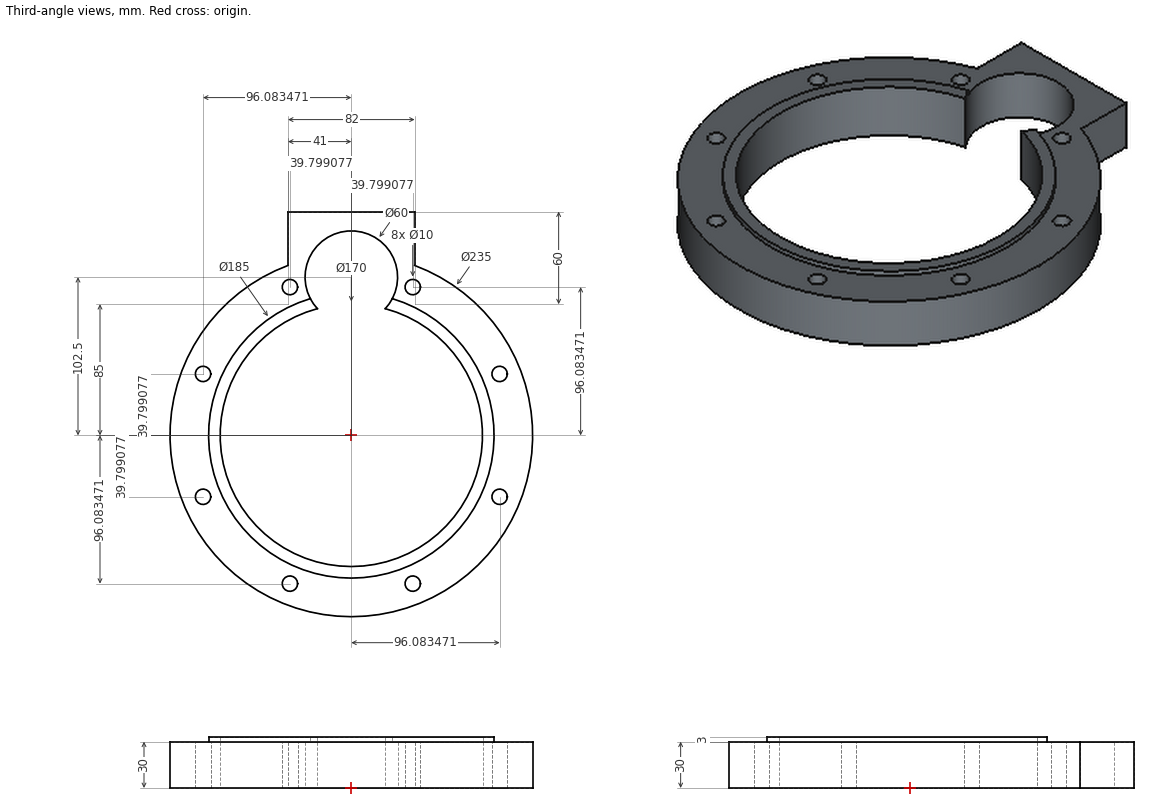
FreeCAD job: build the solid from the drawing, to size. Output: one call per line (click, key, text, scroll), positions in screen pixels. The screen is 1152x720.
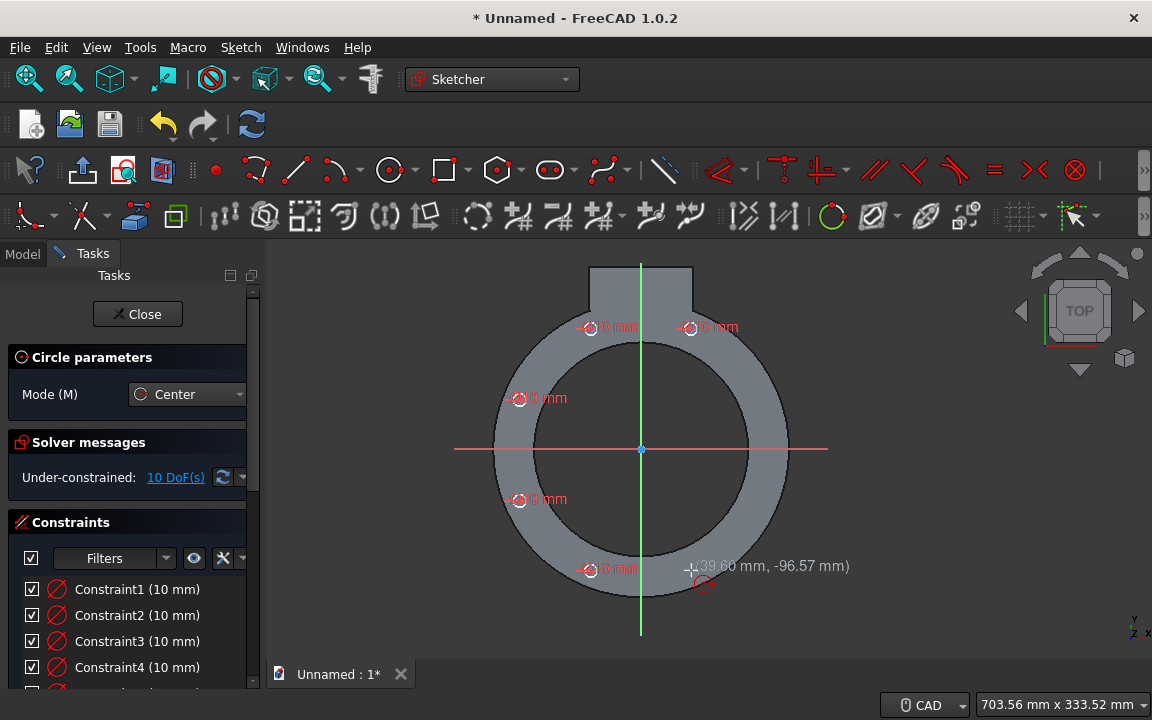
click(691, 570)
move(696, 566)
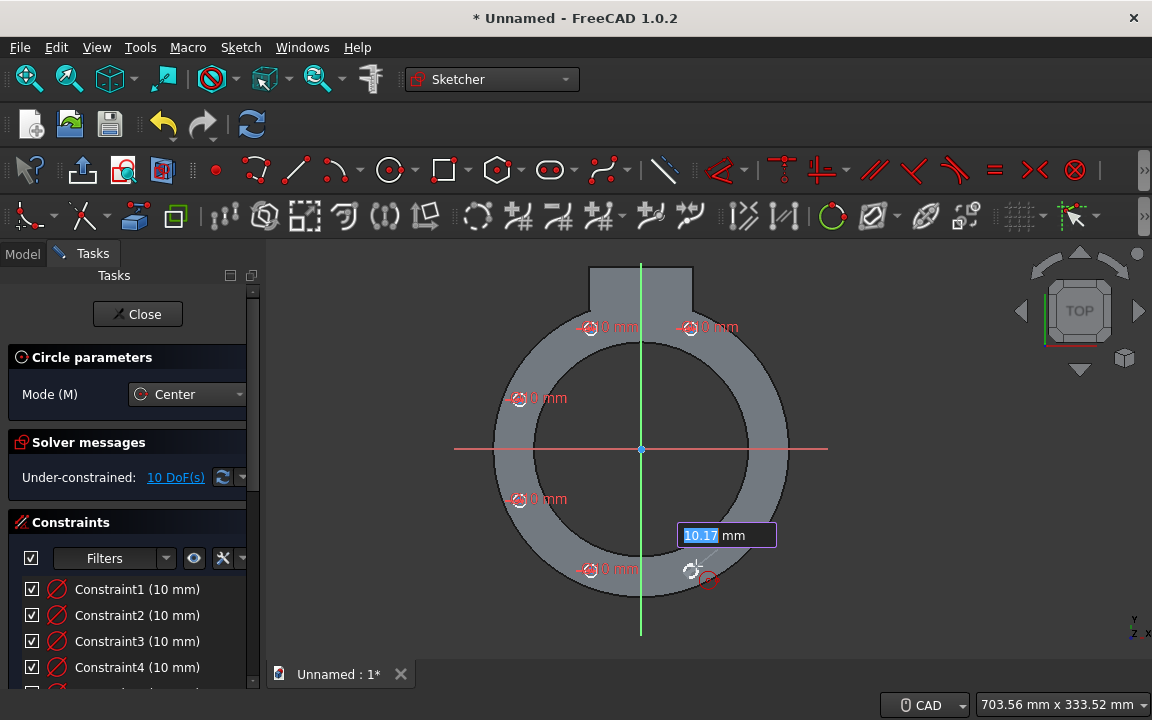
text(10)
key(Return)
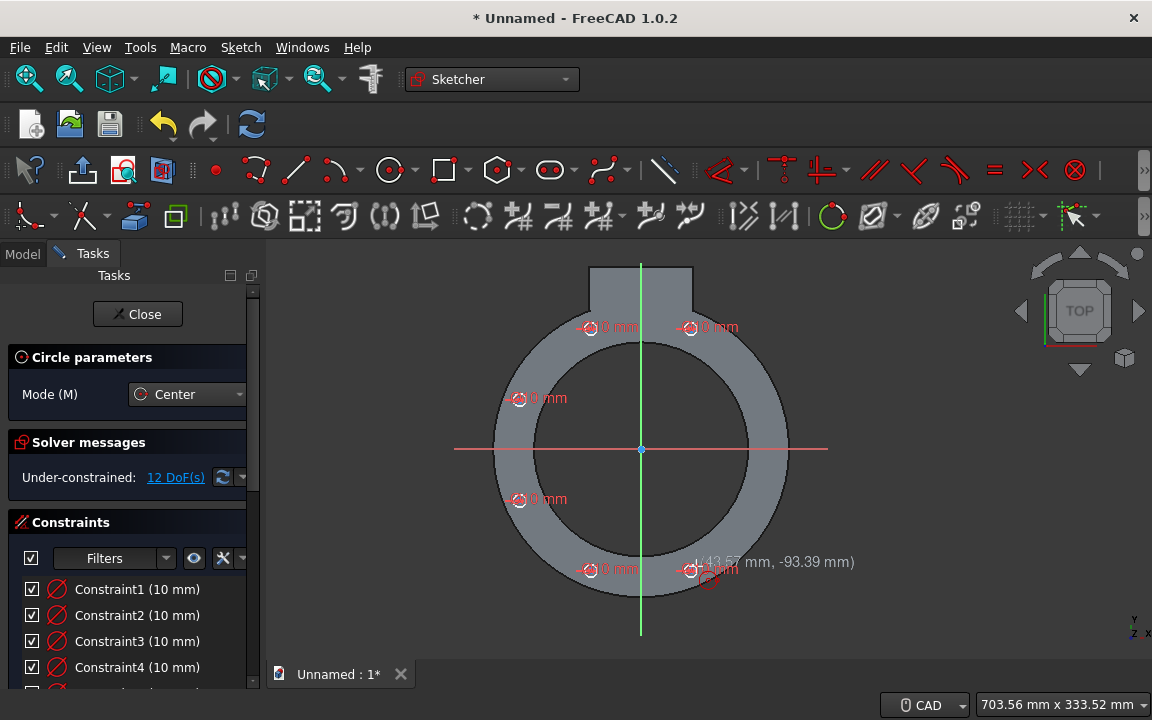
scroll(762, 500, up, 7)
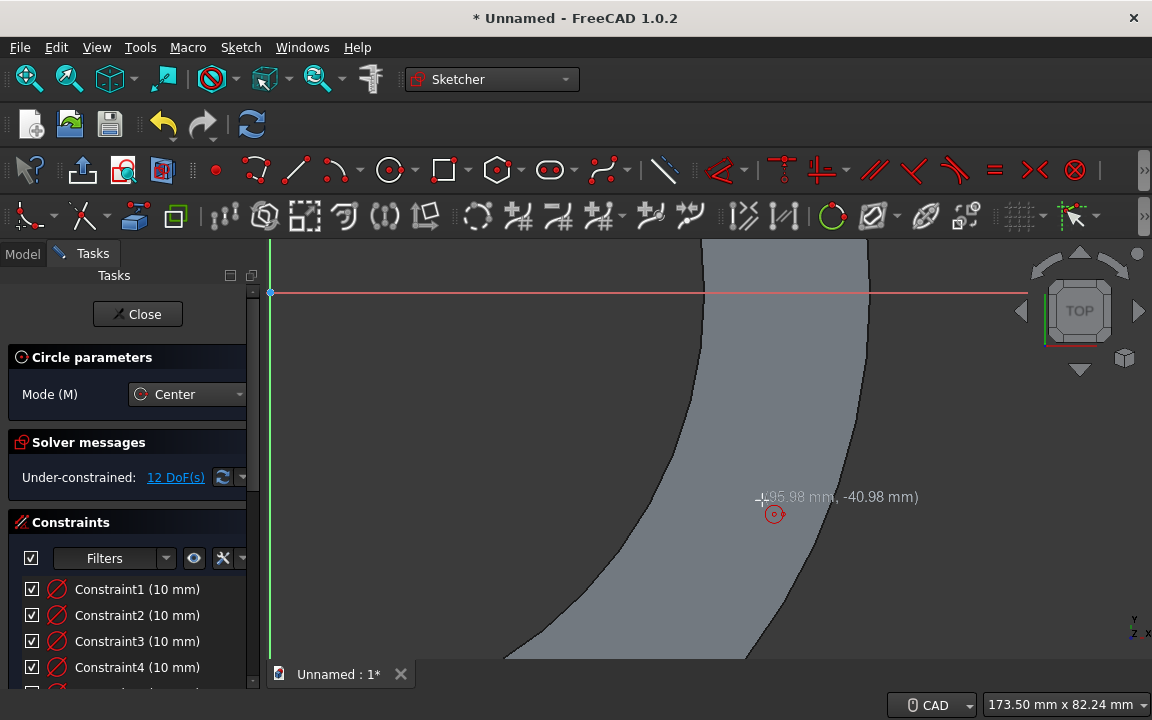
scroll(762, 500, down, 7)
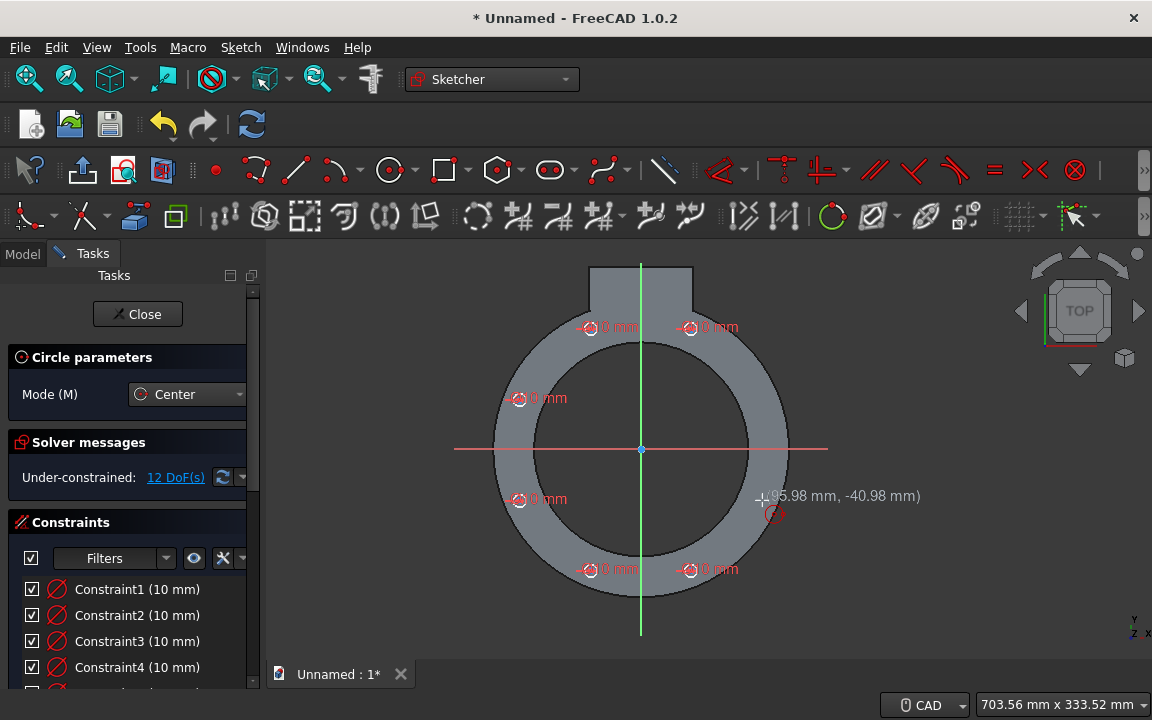
click(762, 500)
move(767, 495)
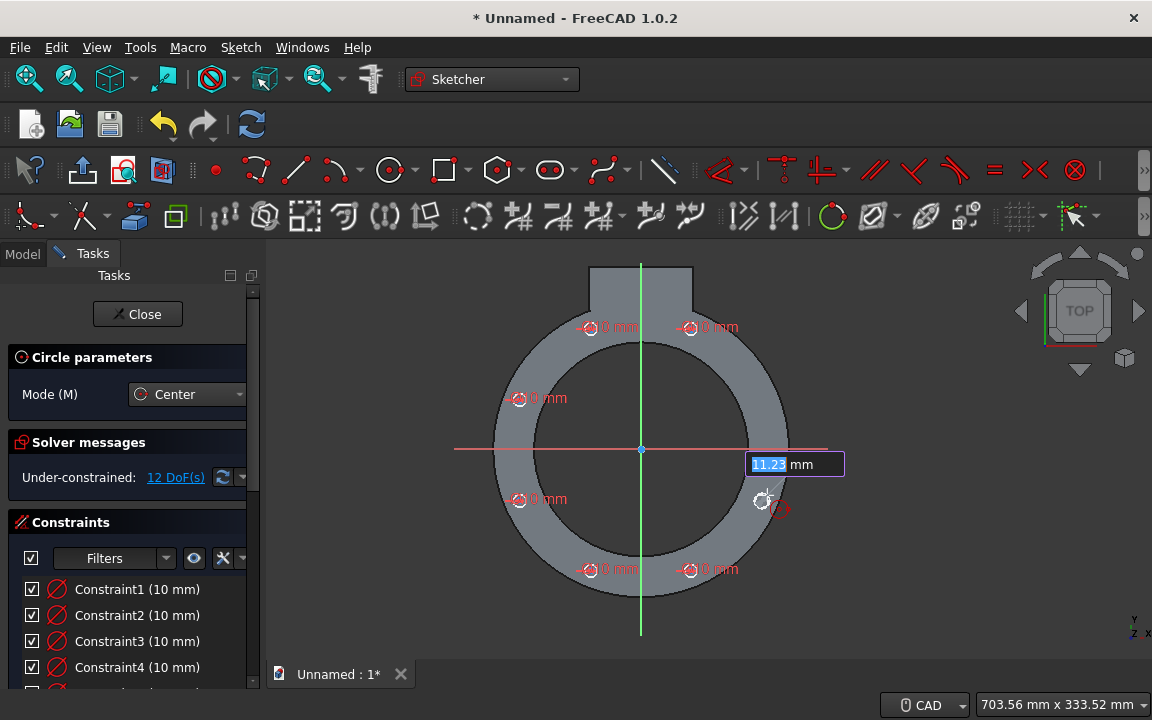
text(10)
key(Return)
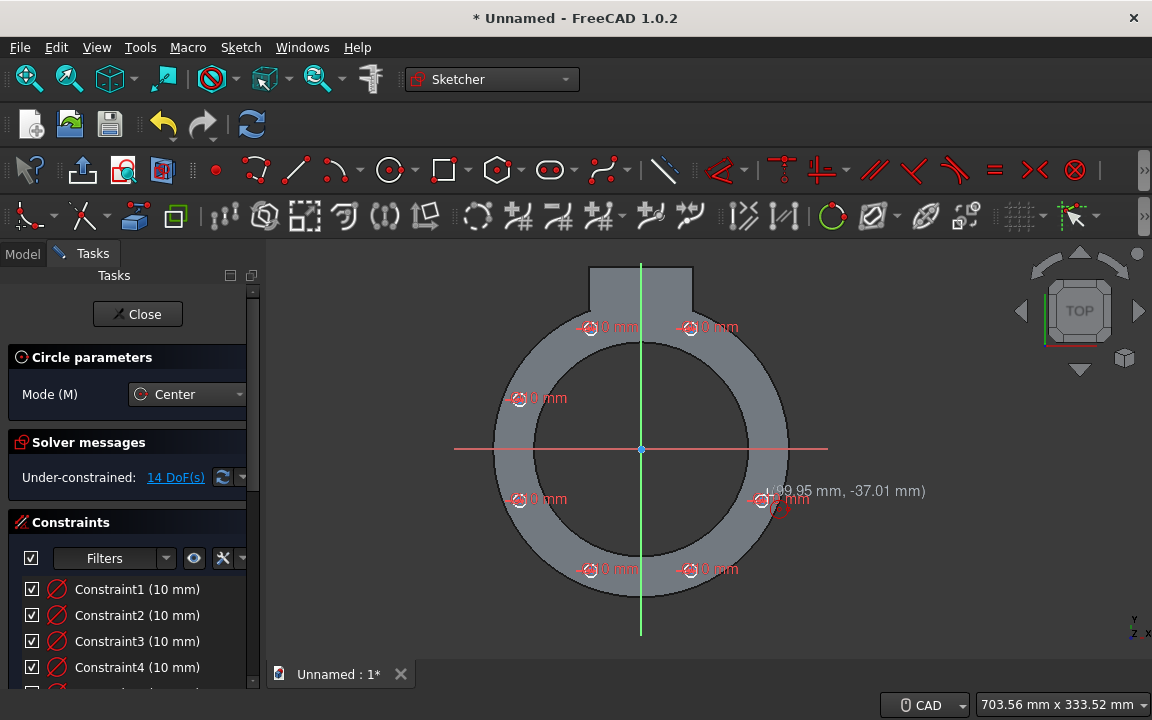
scroll(762, 399, up, 7)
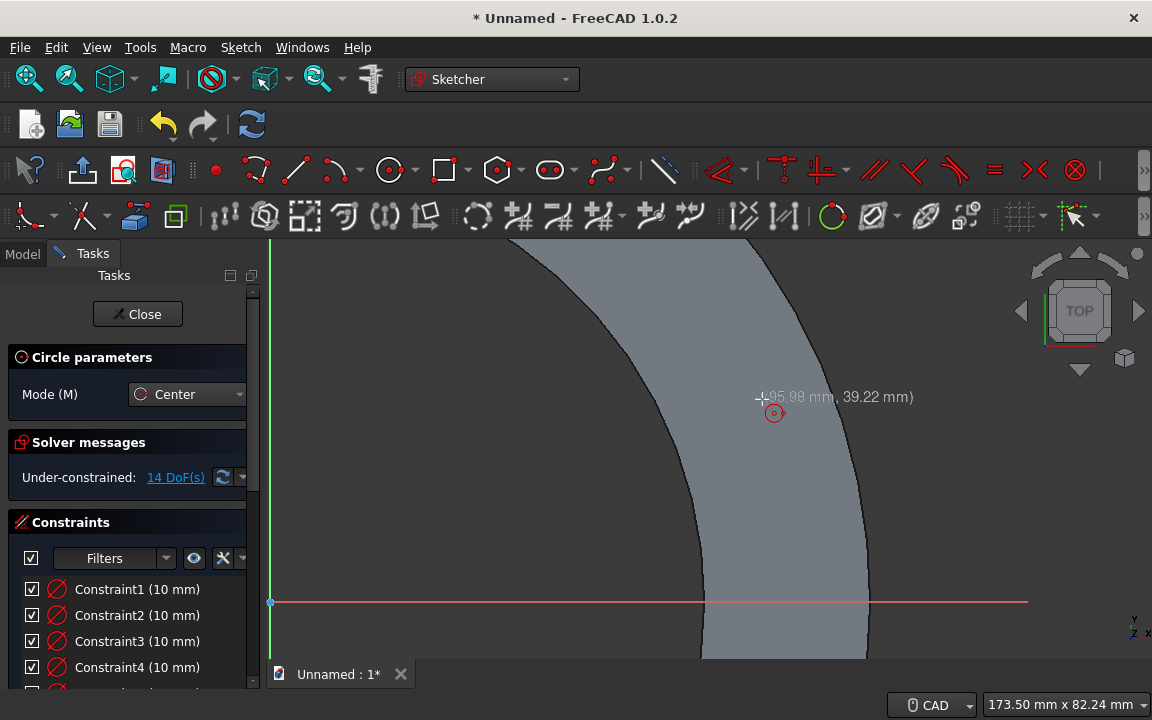
scroll(762, 399, down, 7)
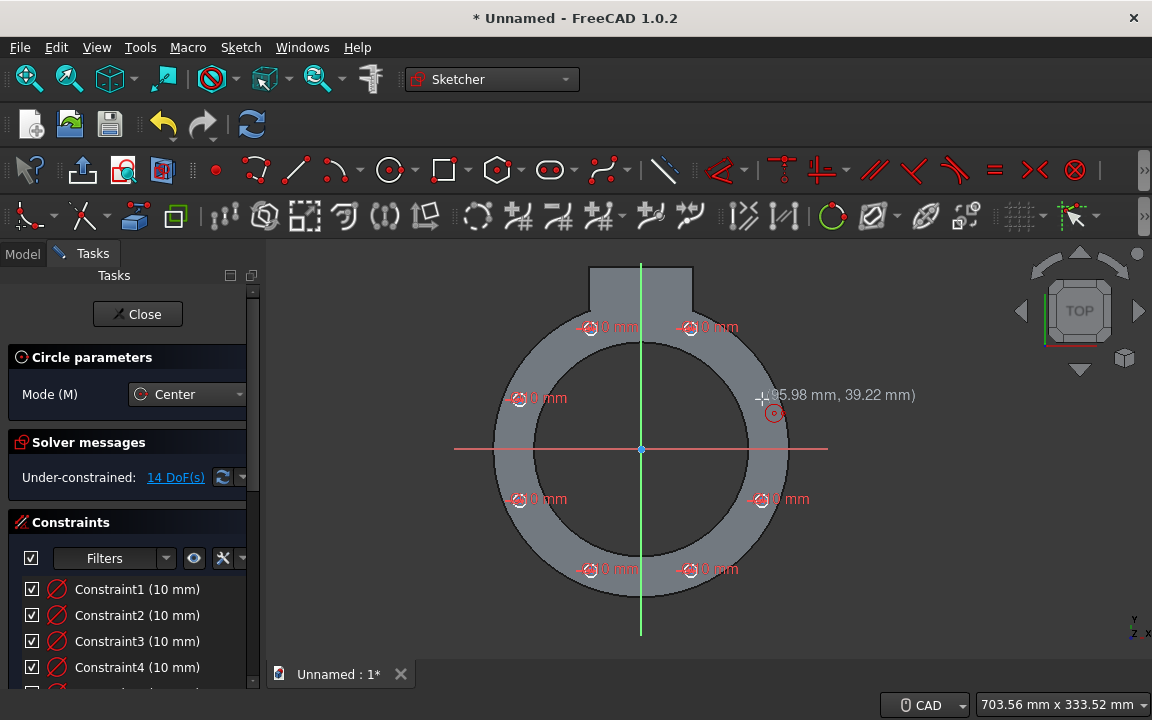
click(762, 399)
move(767, 395)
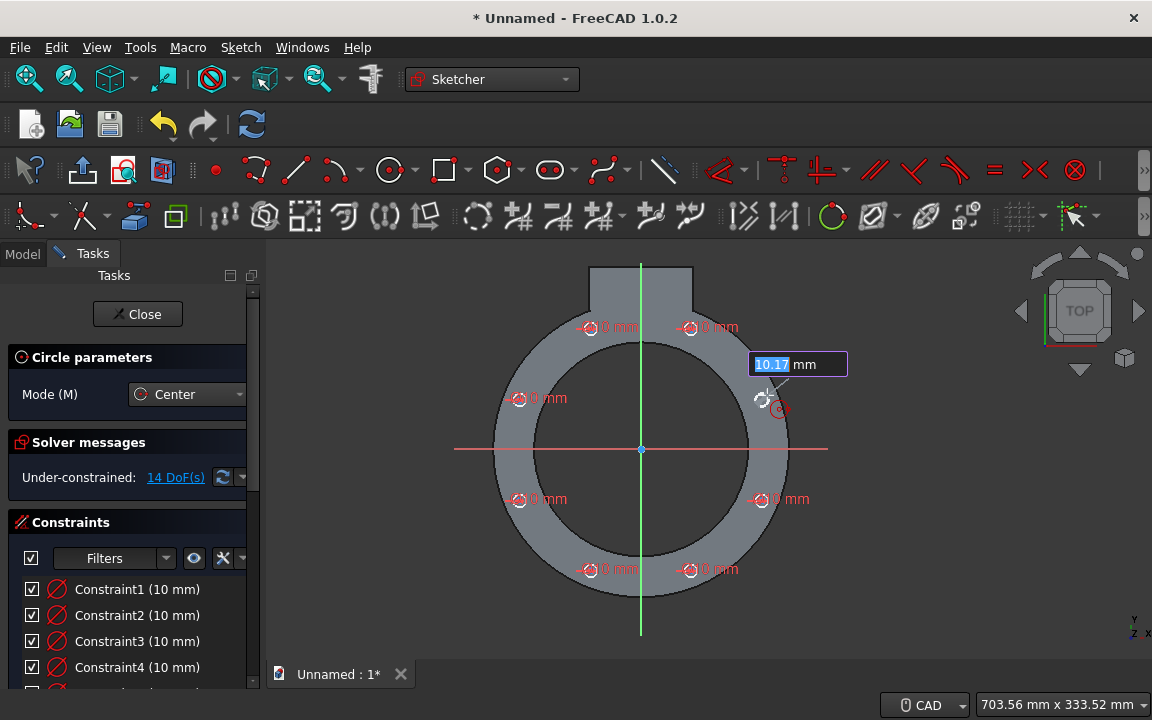
text(10)
key(Return)
key(Escape)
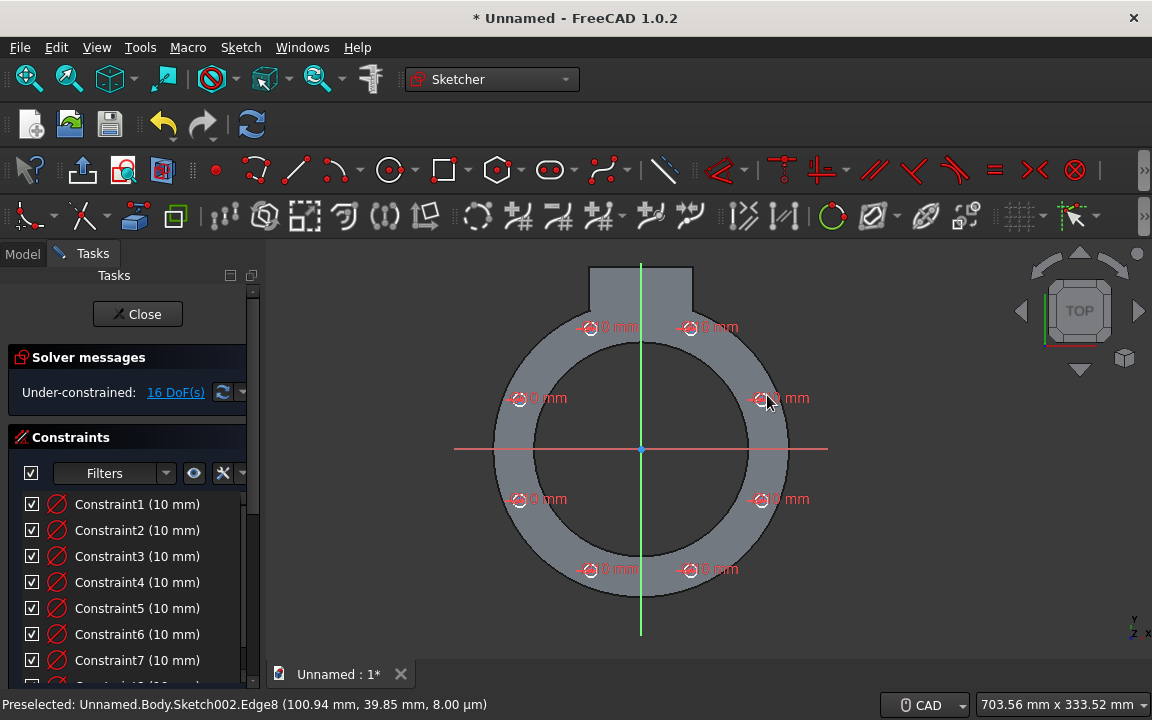
click(691, 329)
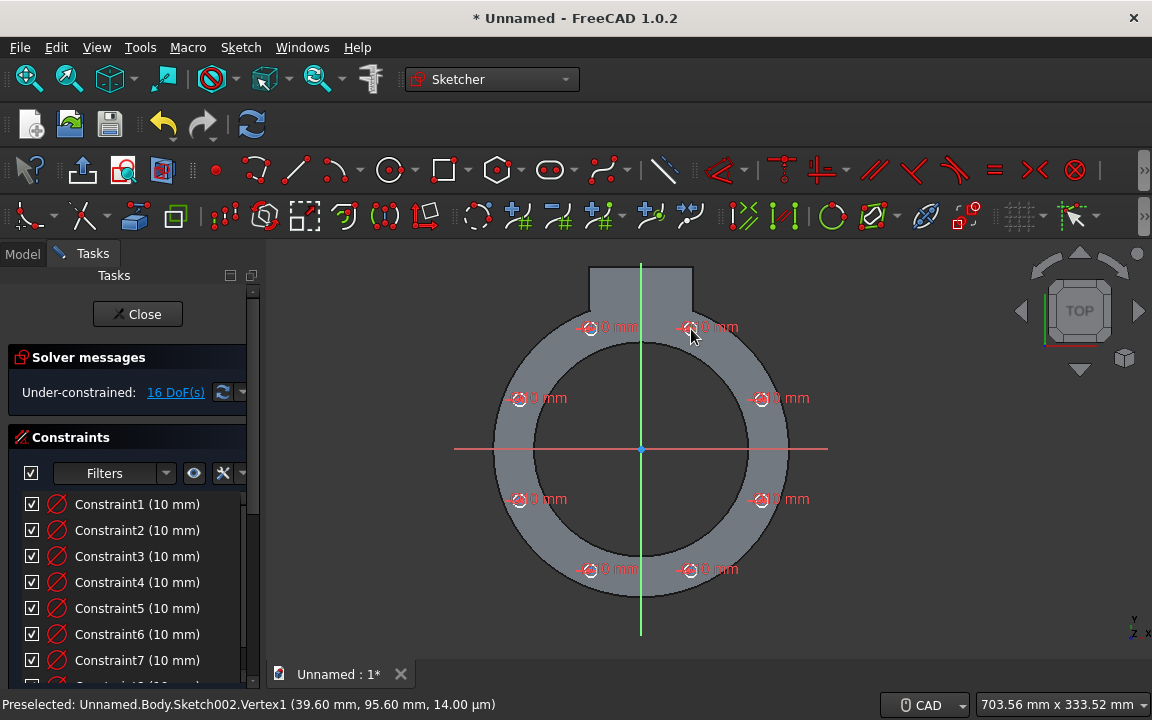
click(591, 329)